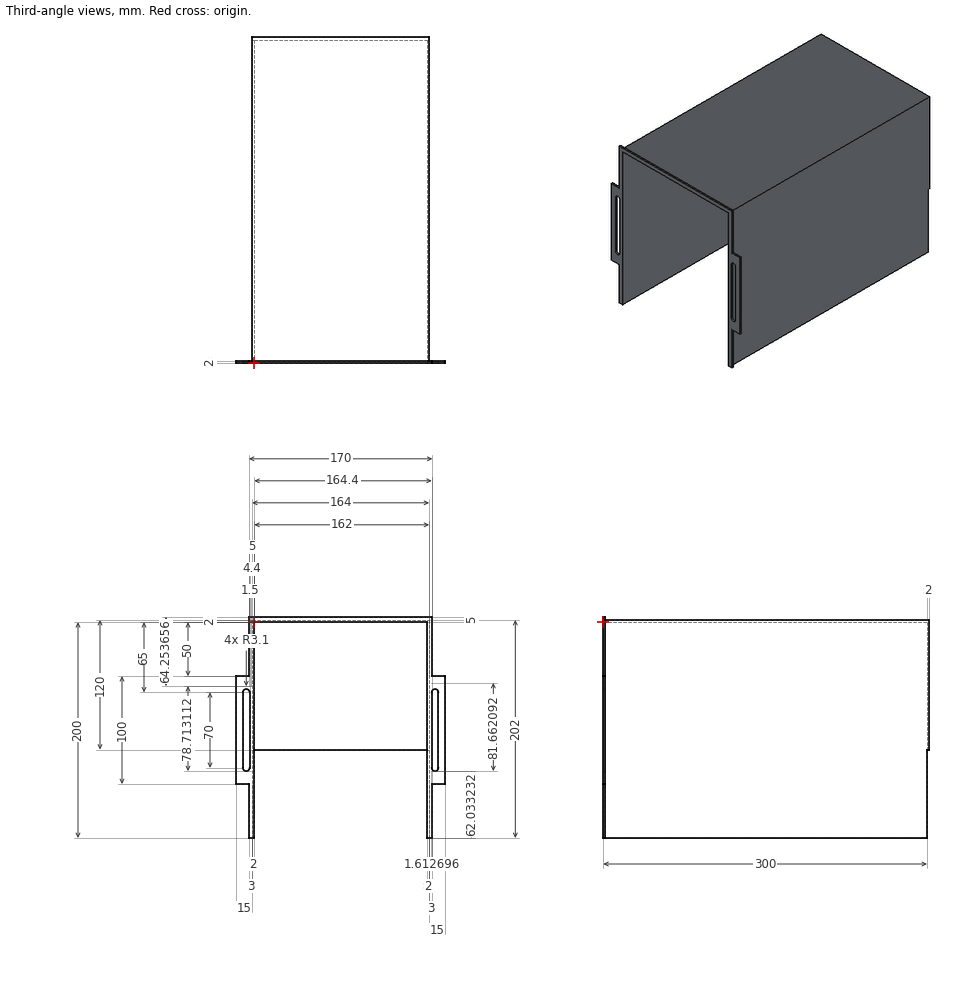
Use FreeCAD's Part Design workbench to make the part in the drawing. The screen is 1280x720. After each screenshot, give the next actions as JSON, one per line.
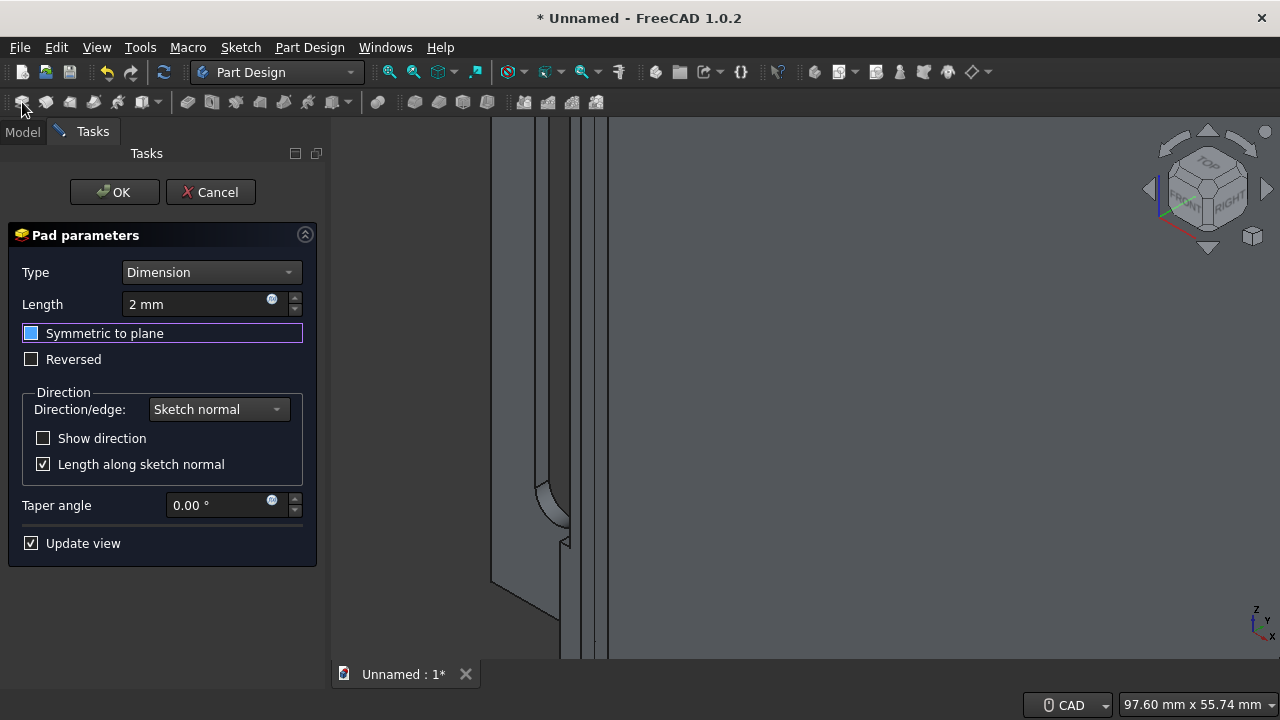
{"action": "left_click", "coordinate": [30, 359]}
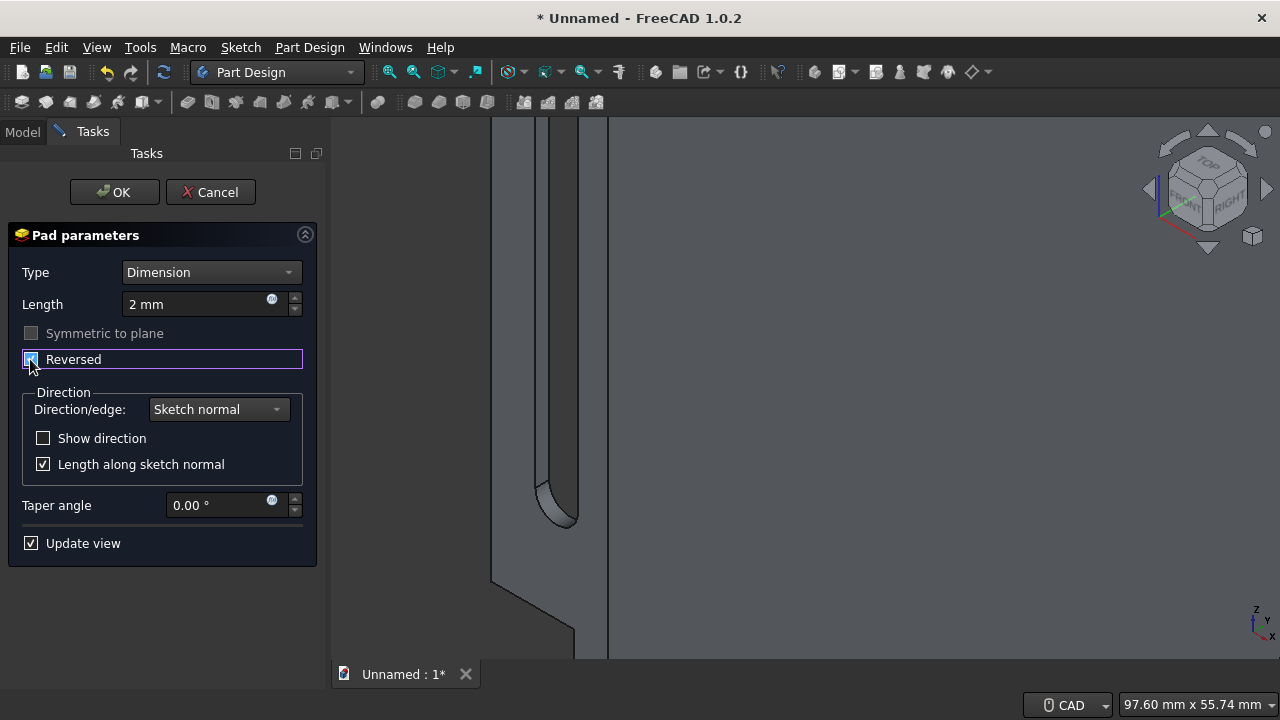
{"action": "left_click", "coordinate": [115, 192]}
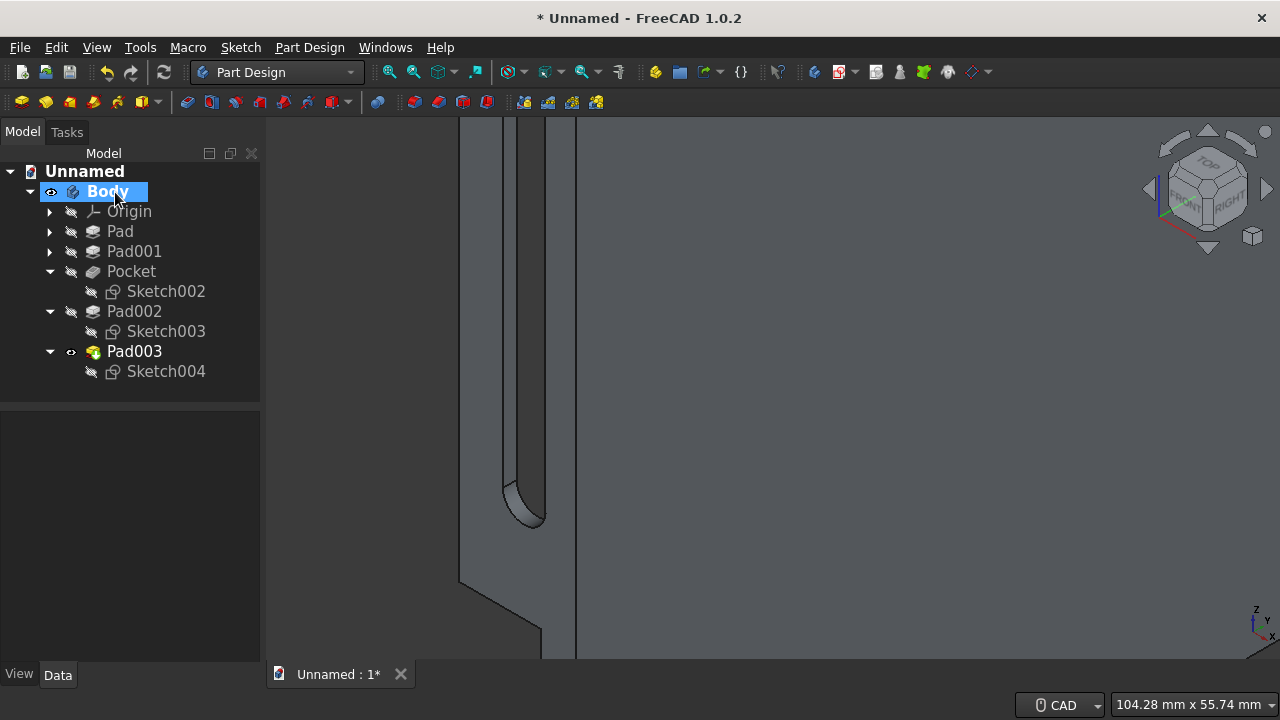
{"action": "left_click", "coordinate": [390, 72]}